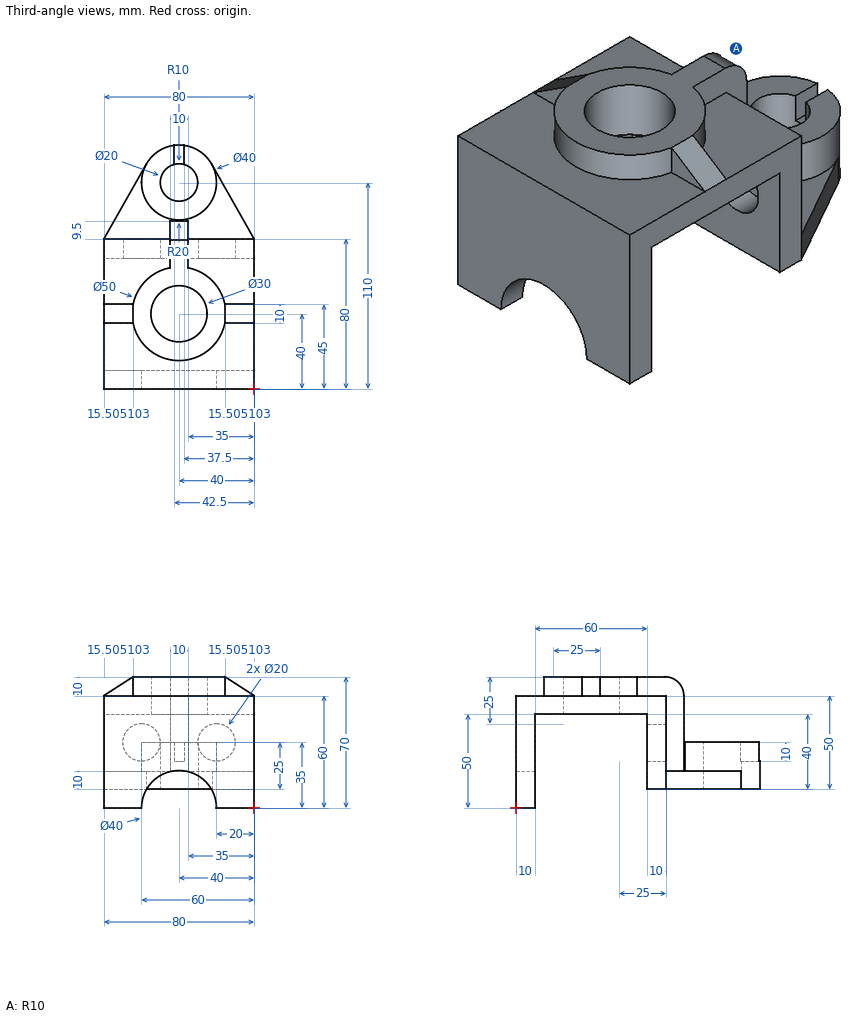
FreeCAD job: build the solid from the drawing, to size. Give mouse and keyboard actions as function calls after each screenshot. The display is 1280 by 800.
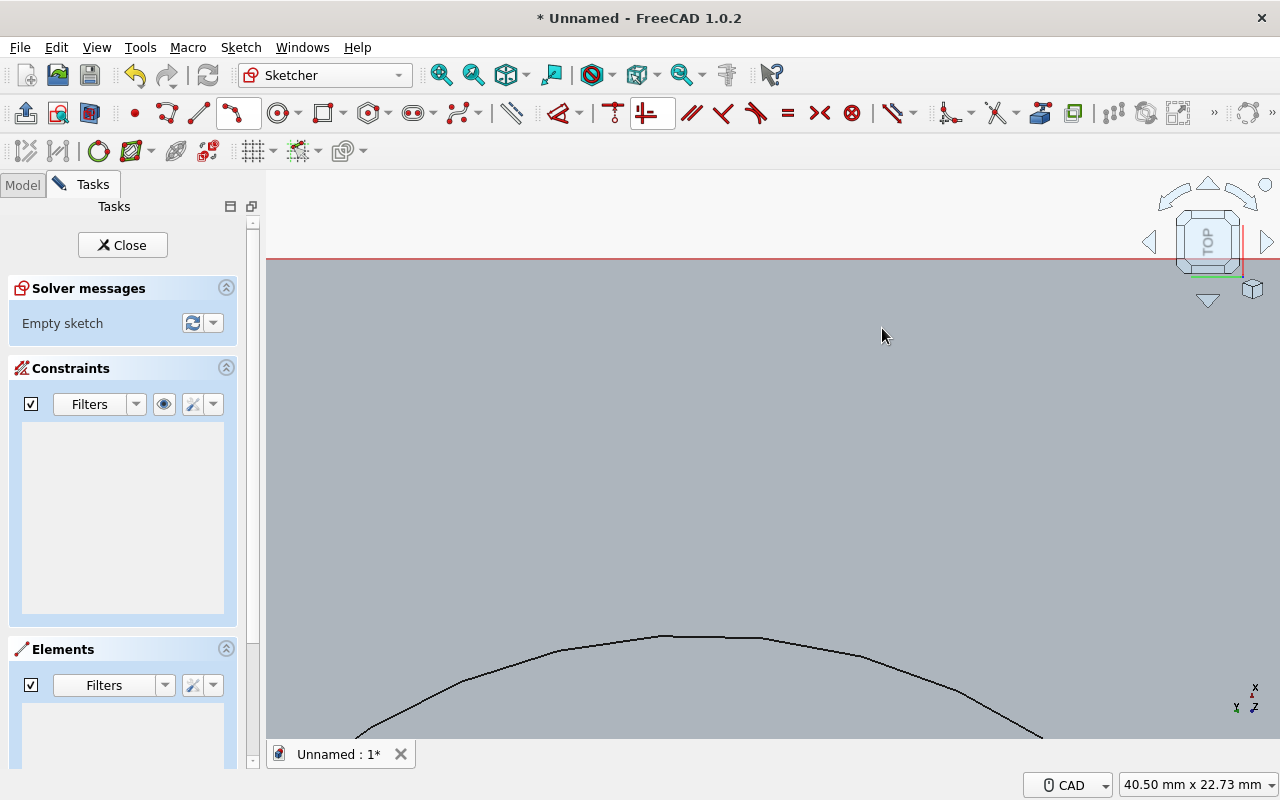
click(324, 114)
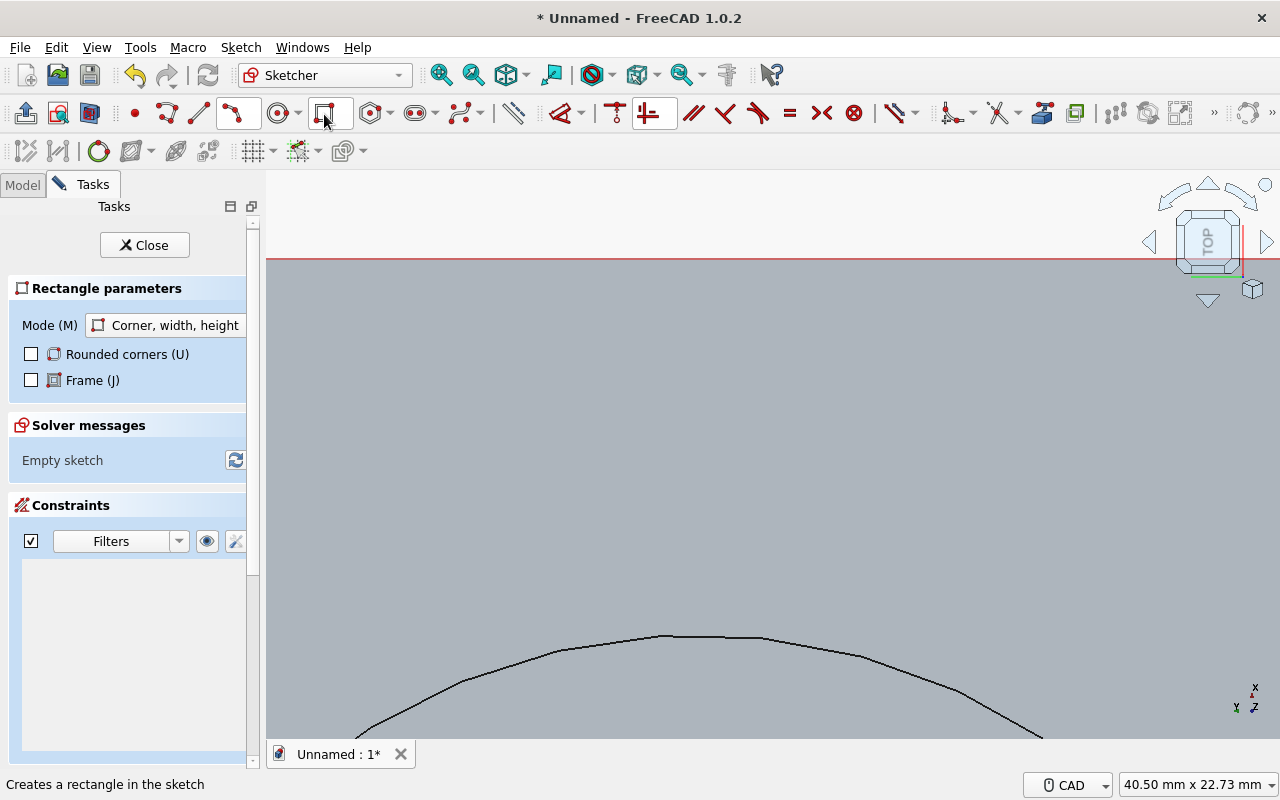
click(573, 259)
move(824, 648)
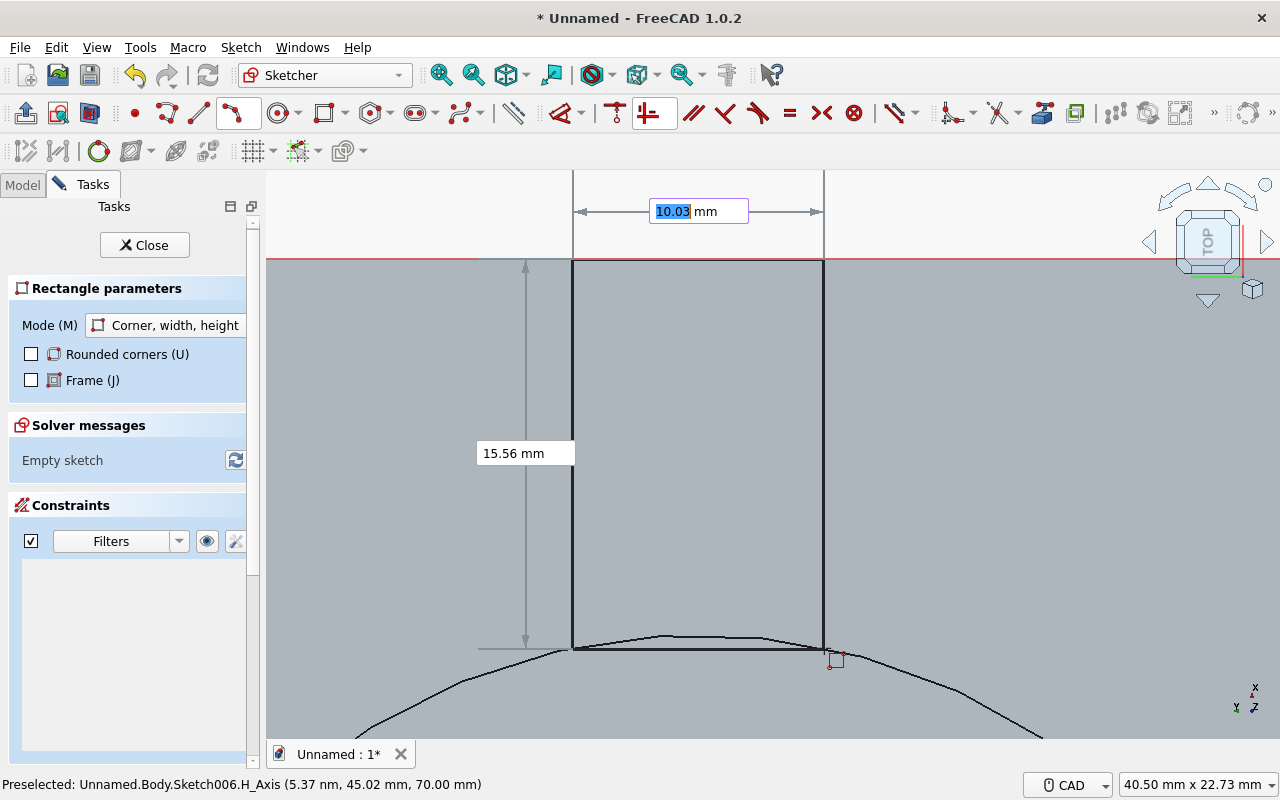
text(10)
key(Tab)
text(15.505103)
key(Return)
key(Escape)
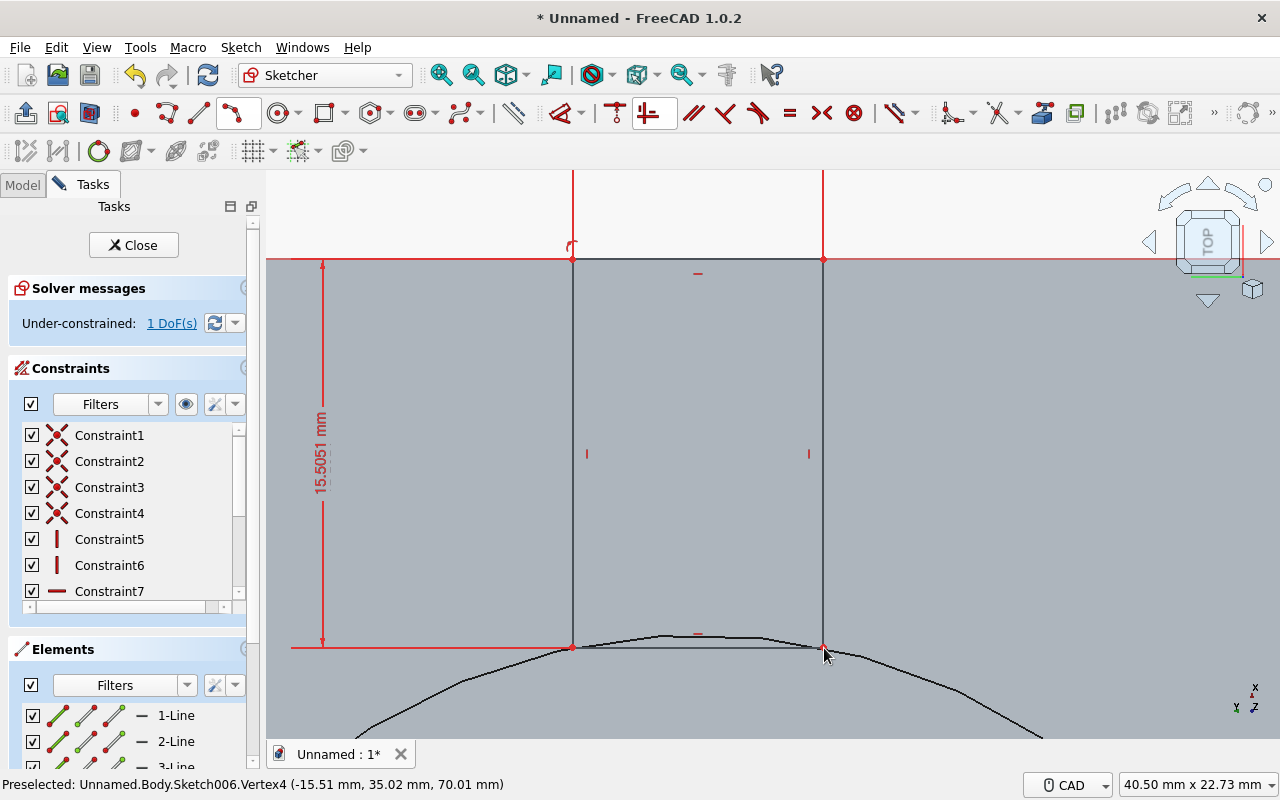
click(560, 114)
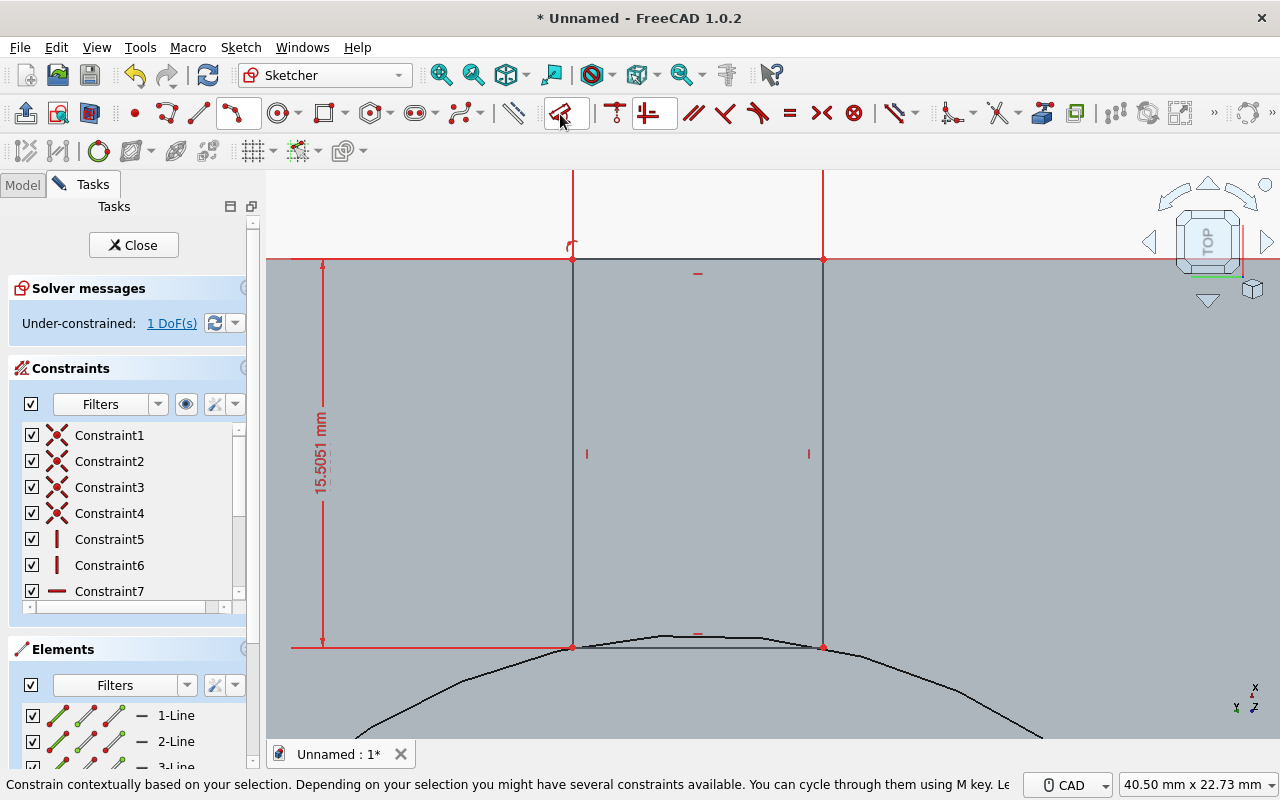
click(573, 259)
click(844, 225)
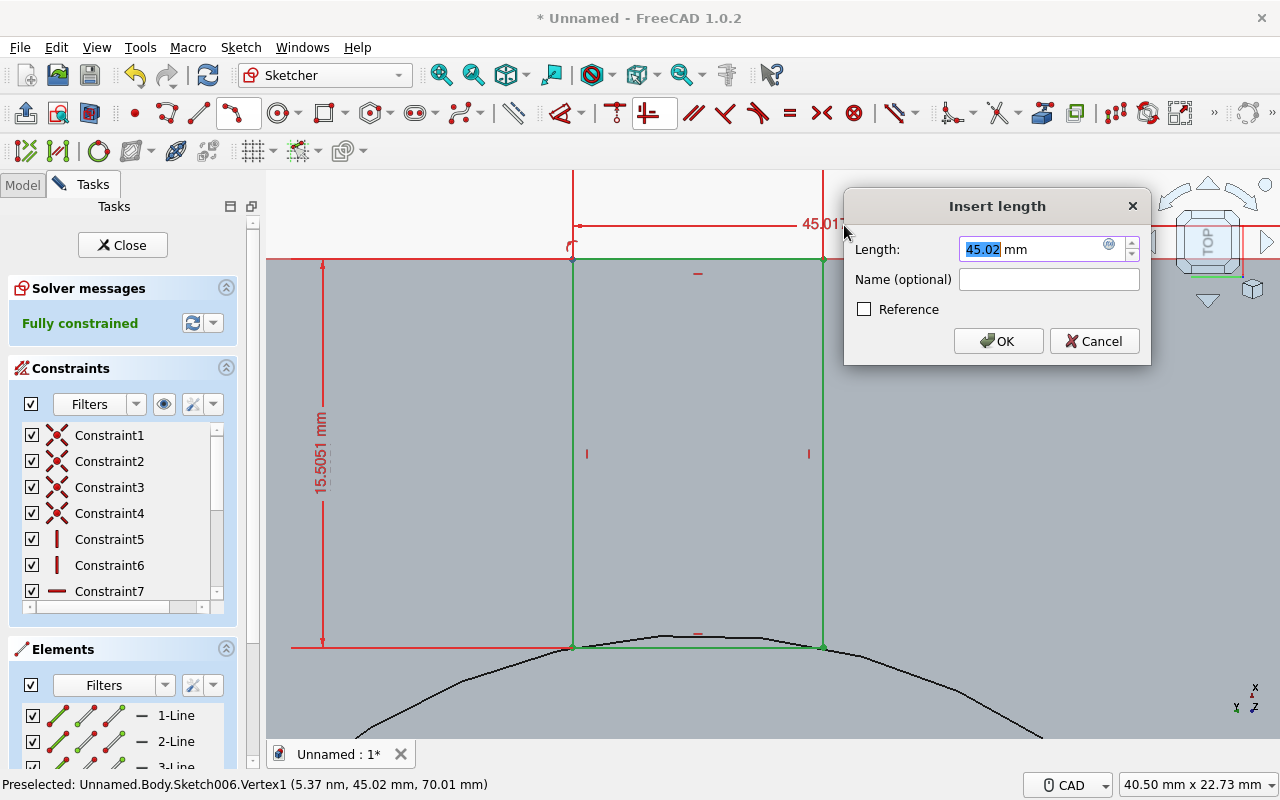
text(45)
key(Return)
key(Escape)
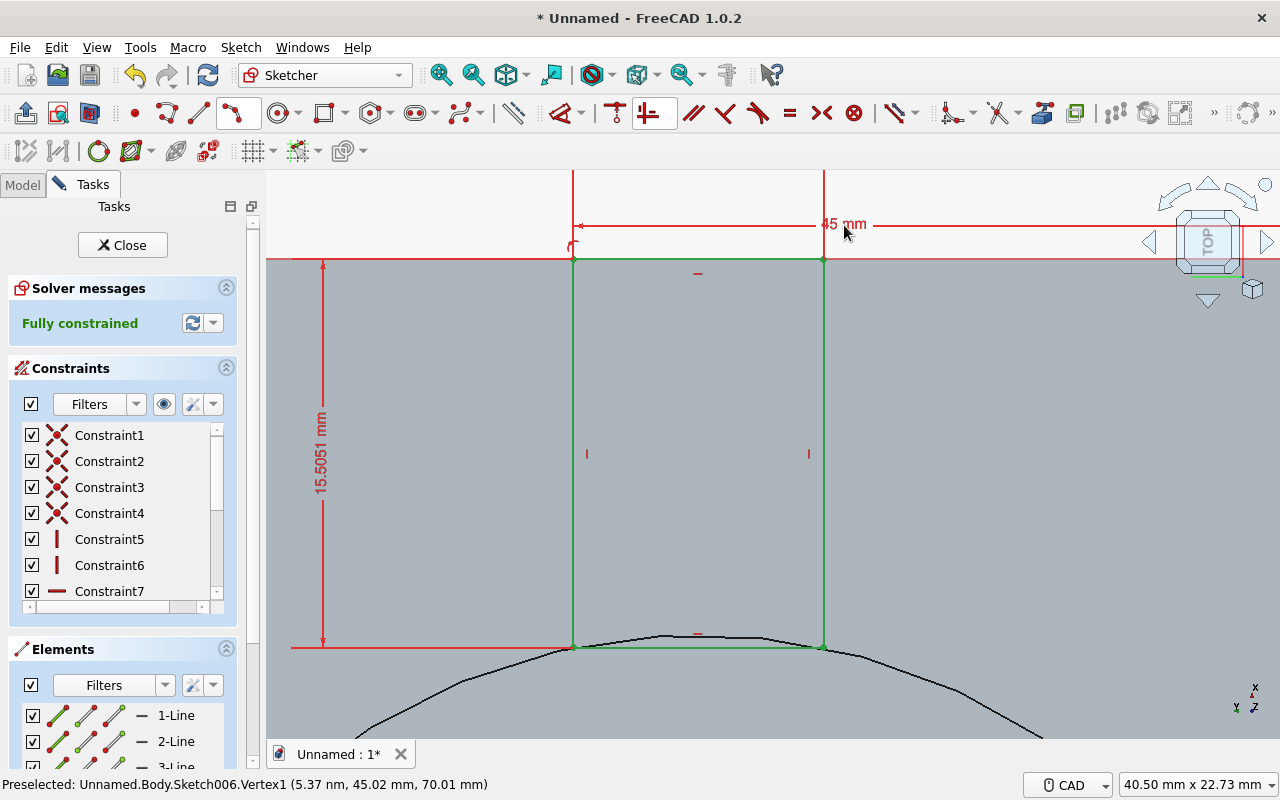
click(123, 245)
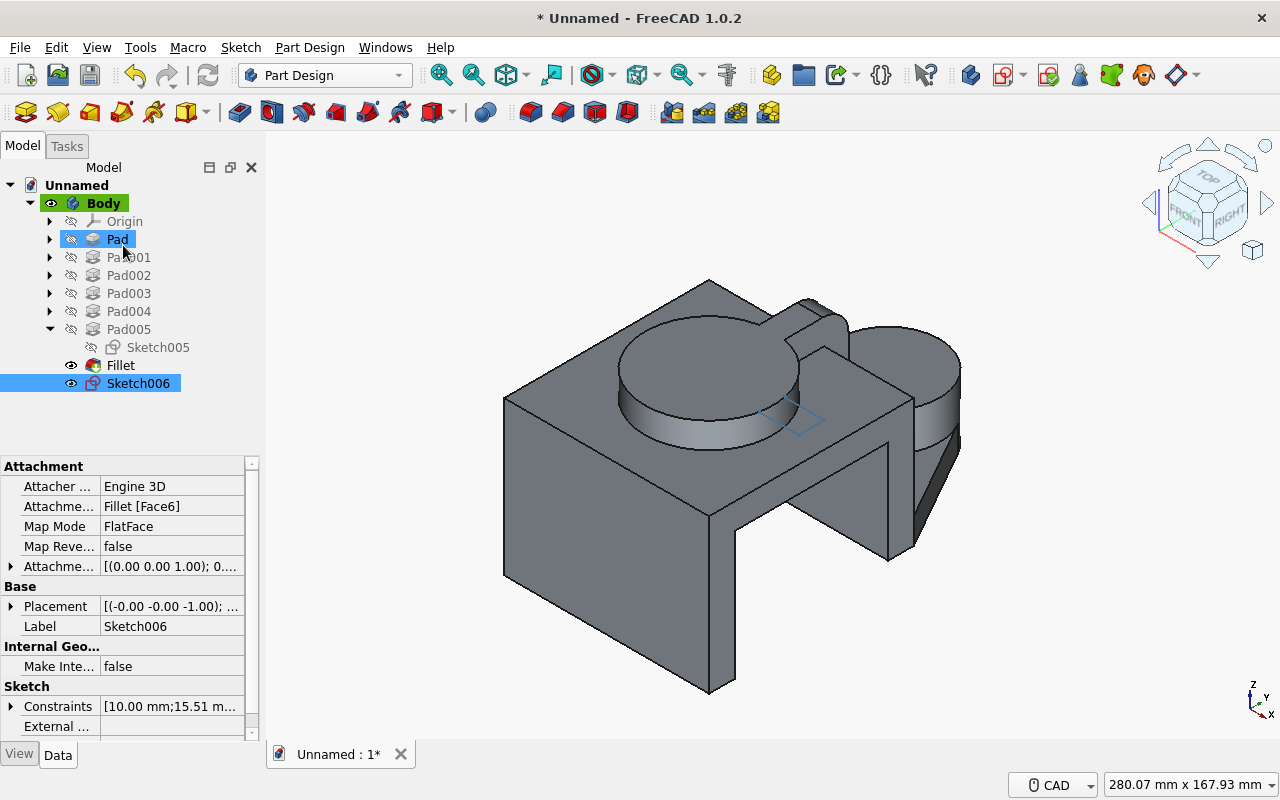
click(26, 112)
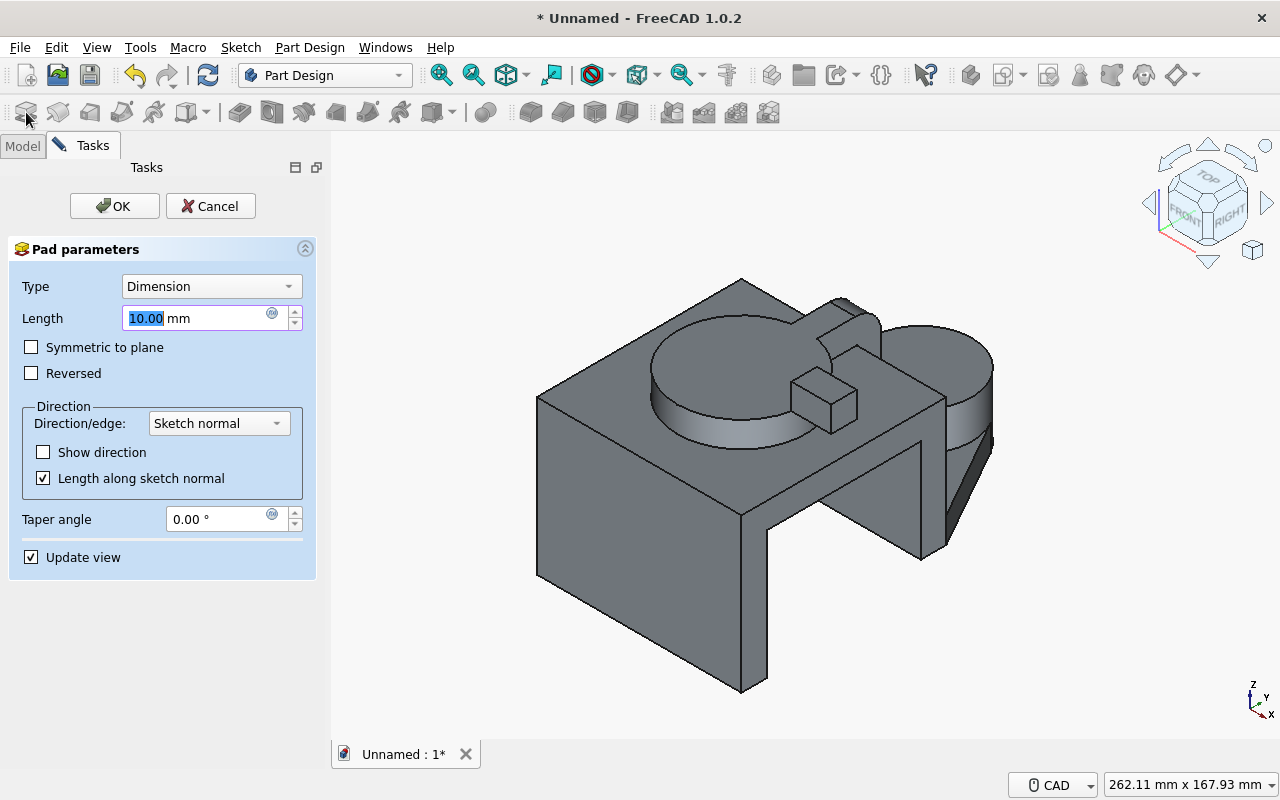
click(212, 286)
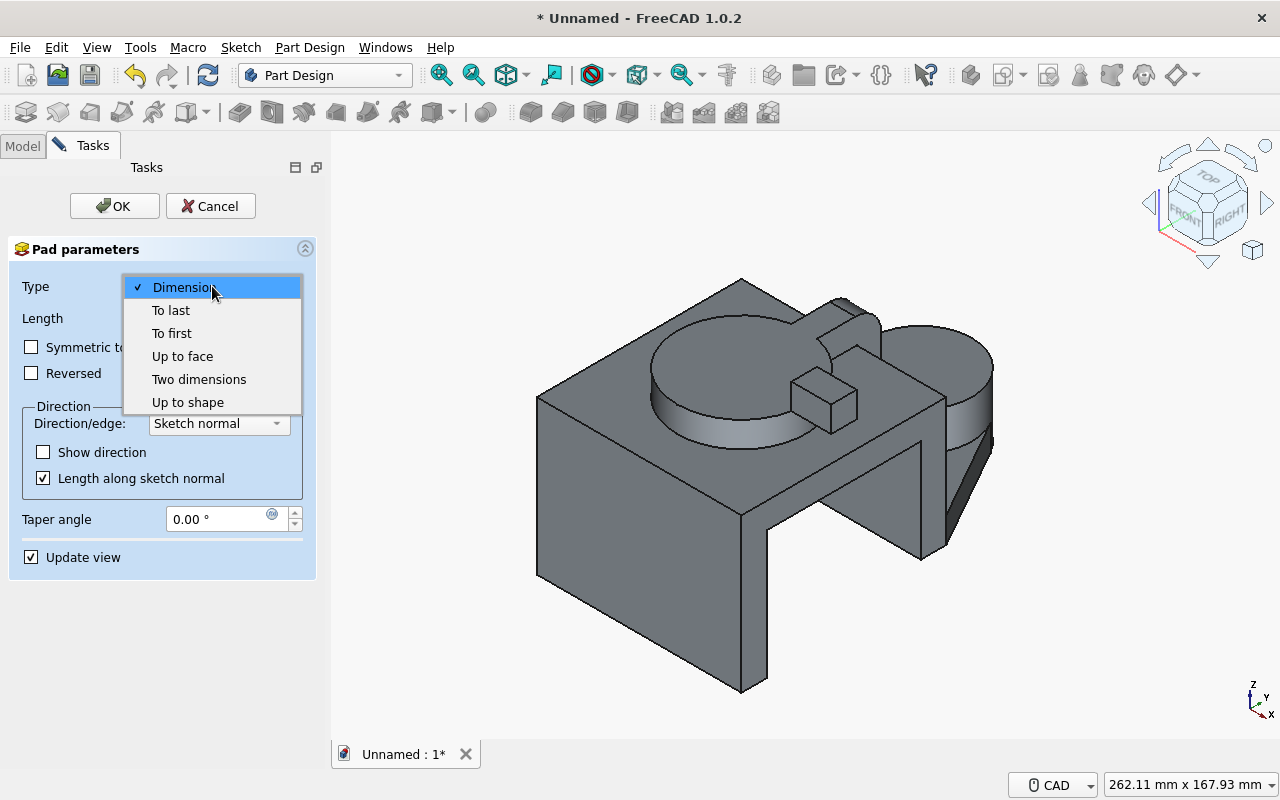
click(212, 334)